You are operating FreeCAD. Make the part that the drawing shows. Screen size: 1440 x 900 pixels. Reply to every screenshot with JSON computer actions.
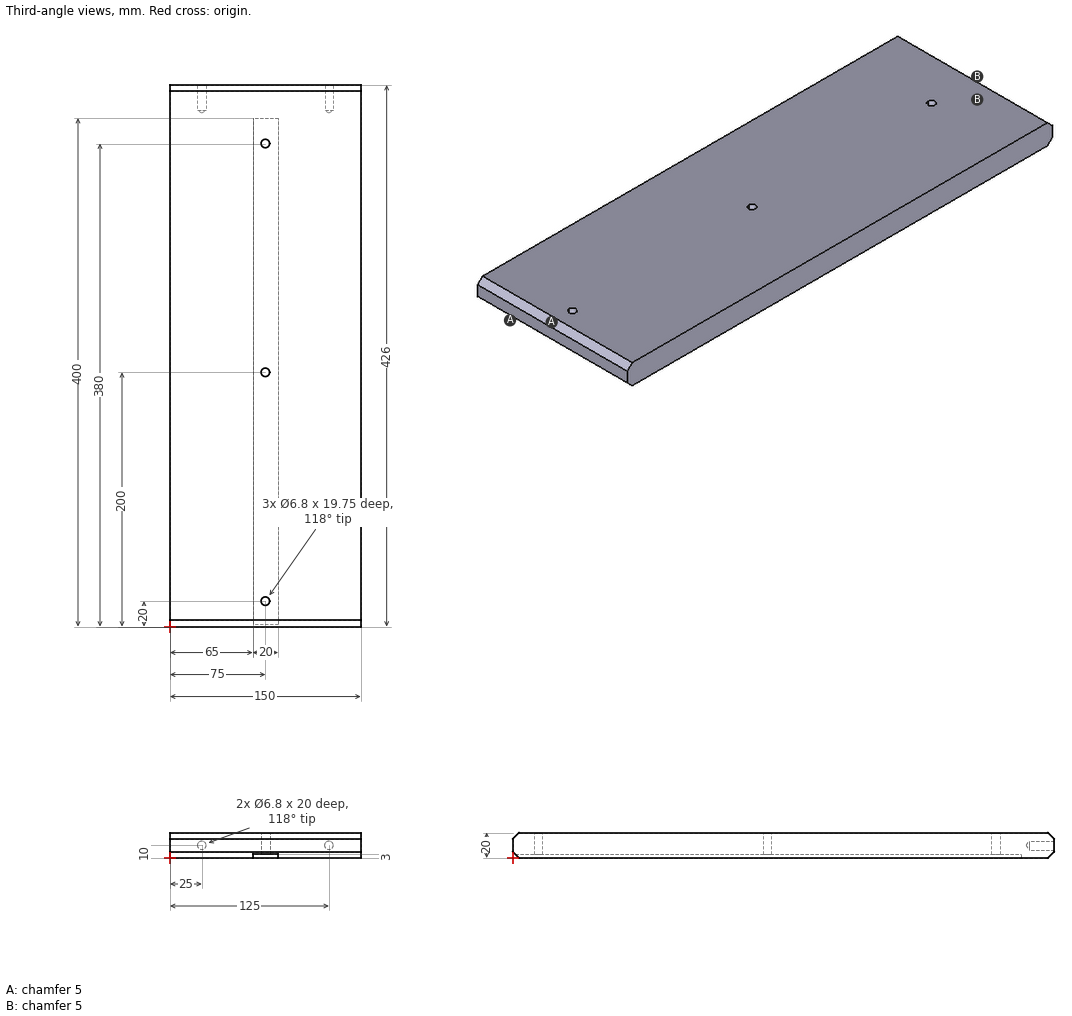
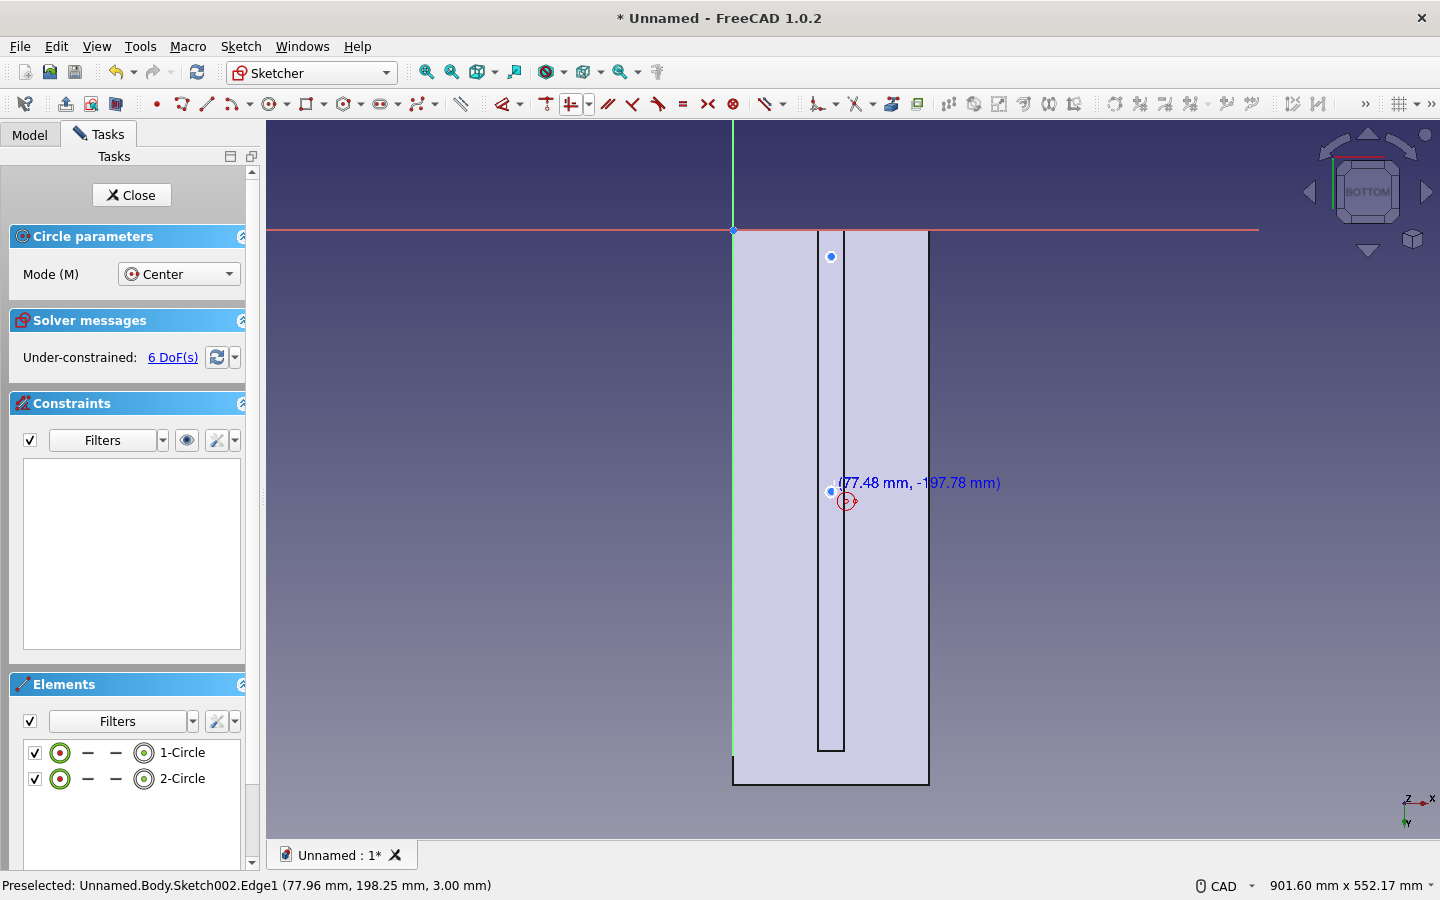
{"action": "scroll", "coordinate": [831, 725], "scroll_direction": "up", "scroll_amount": 9}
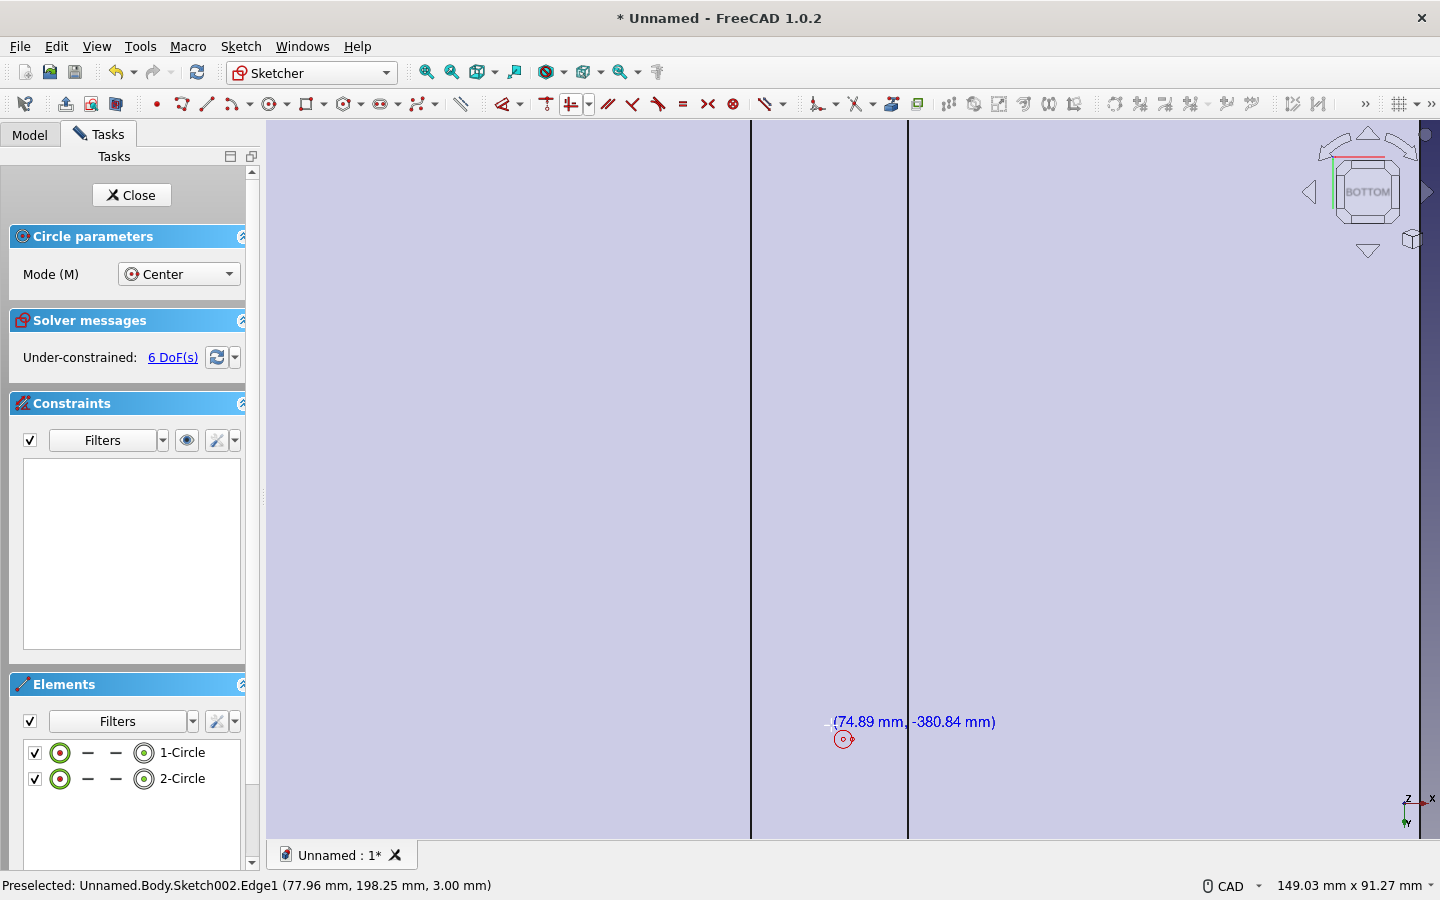
{"action": "scroll", "coordinate": [831, 726], "scroll_direction": "down", "scroll_amount": 9}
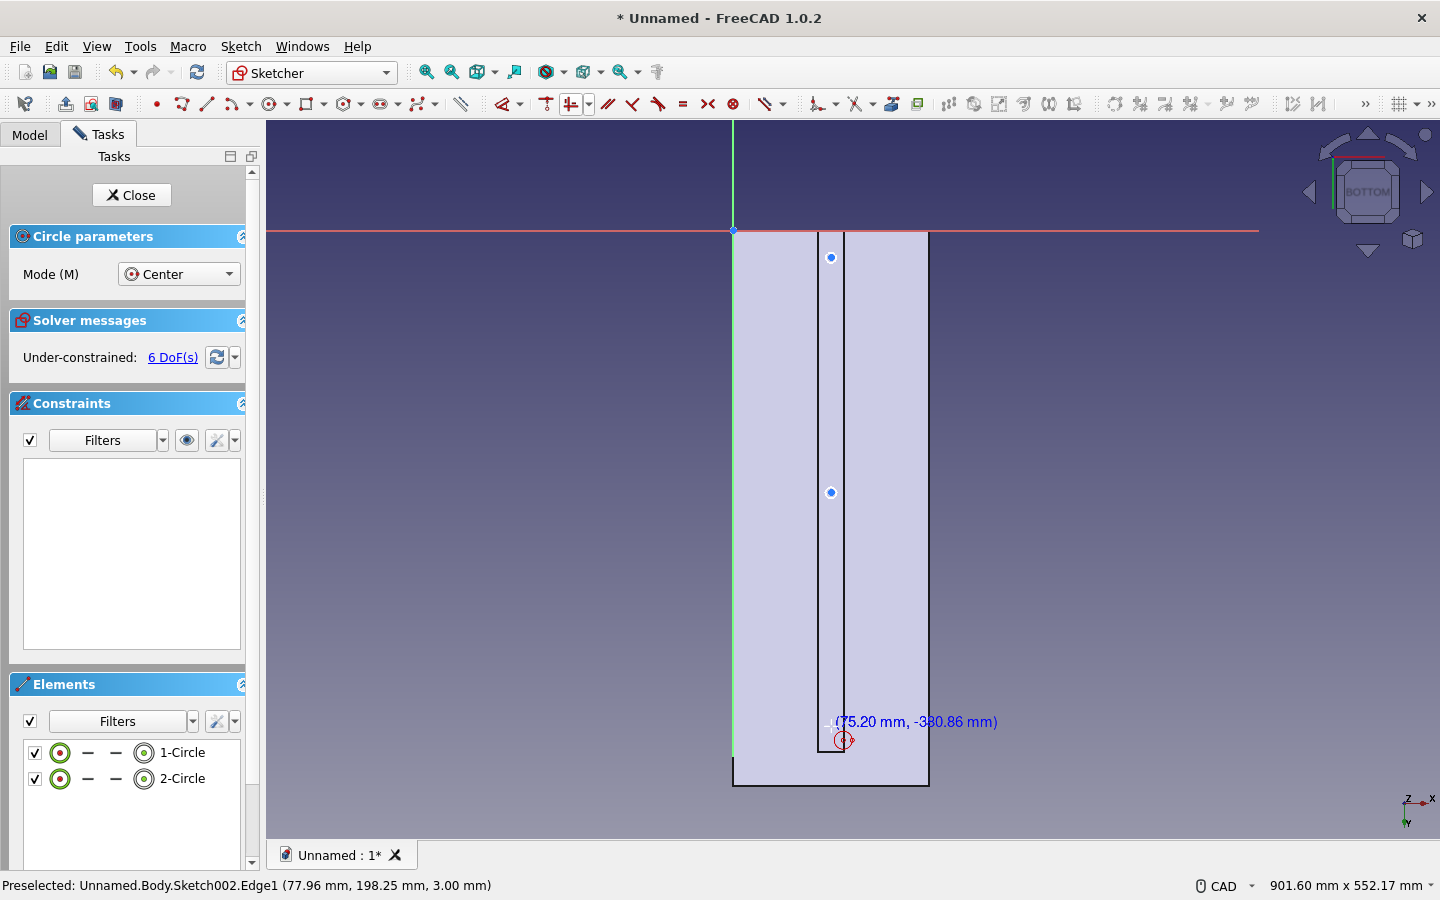
{"action": "left_click", "coordinate": [831, 726]}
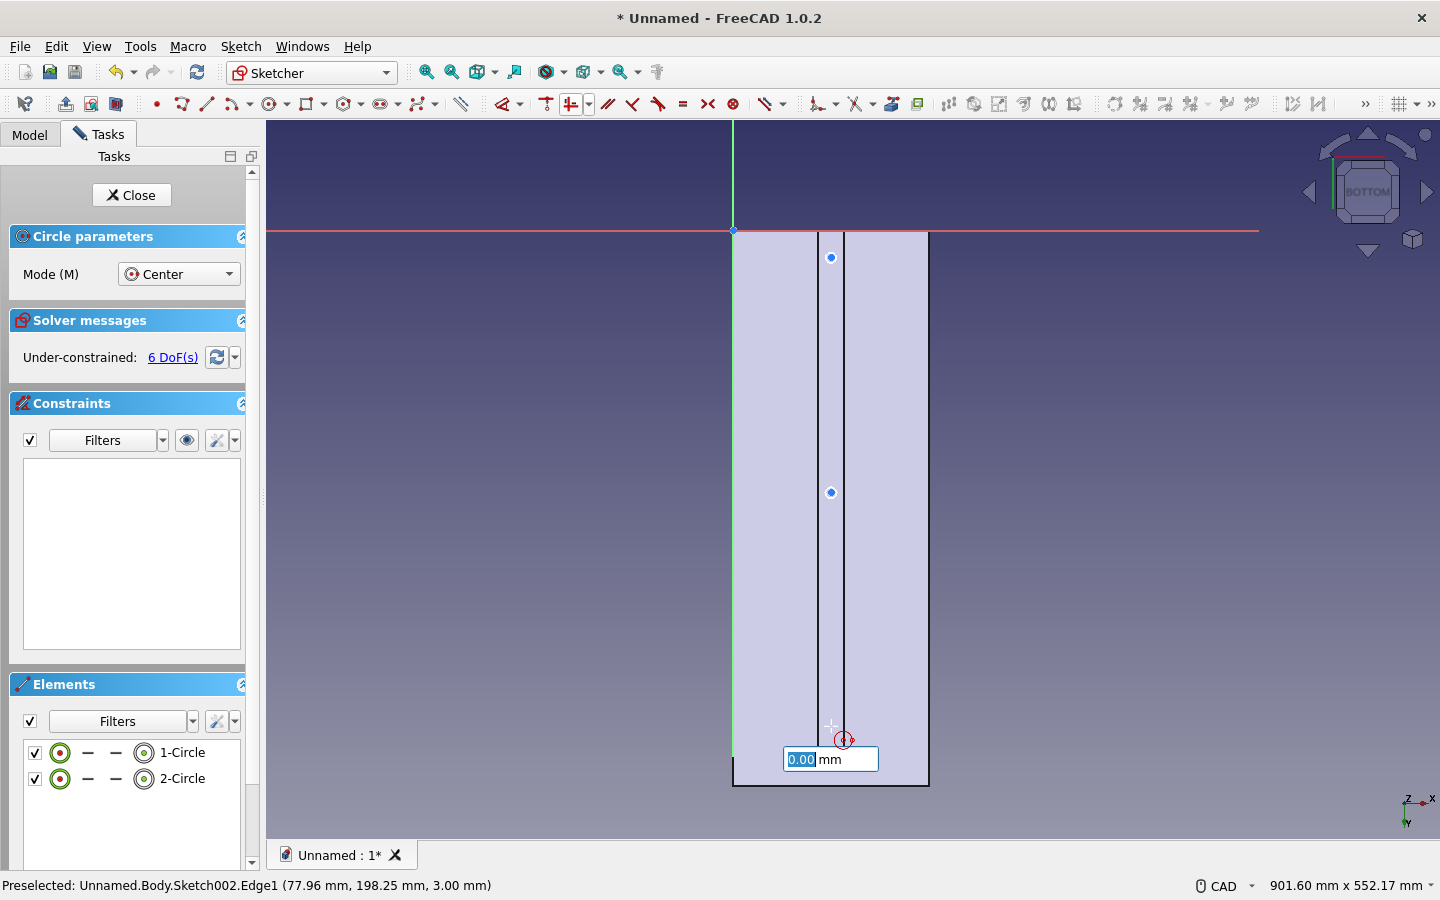
{"action": "scroll", "coordinate": [834, 723], "scroll_direction": "up", "scroll_amount": 7}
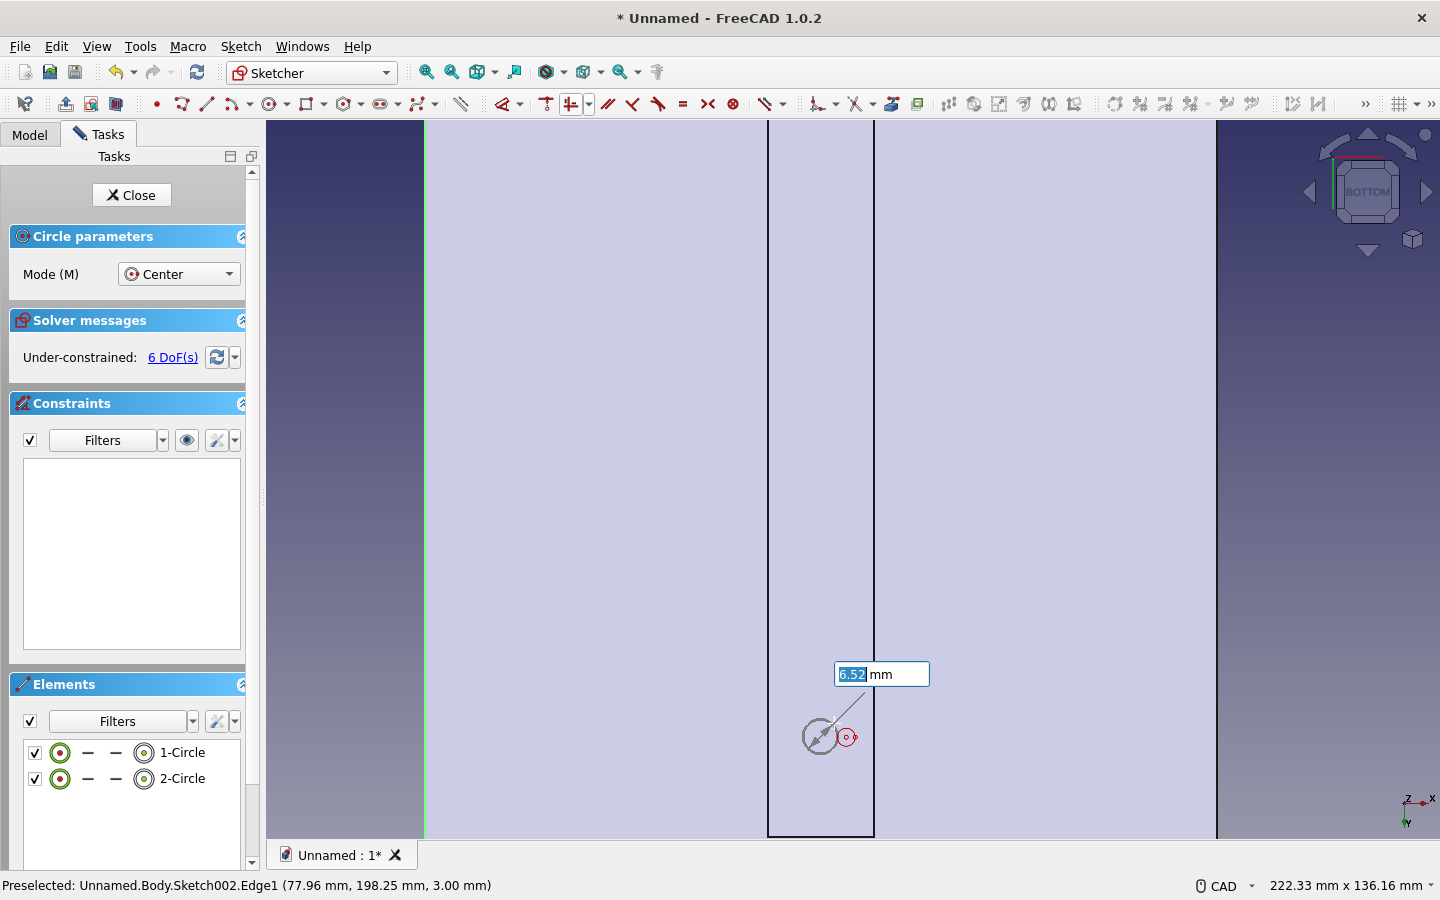
{"action": "left_click", "coordinate": [834, 719]}
{"action": "key", "text": "Escape"}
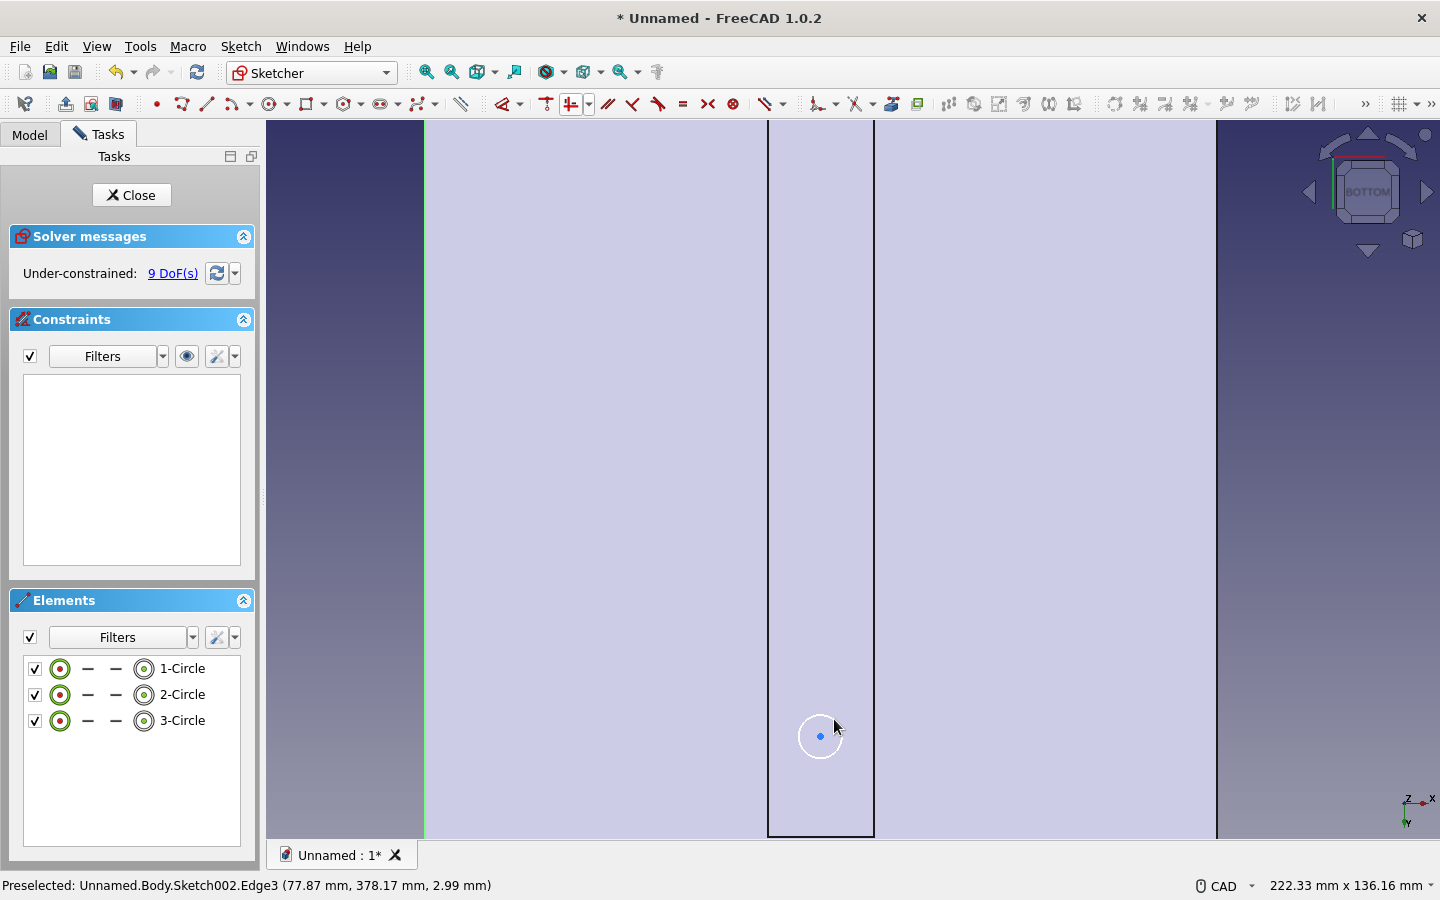
{"action": "scroll", "coordinate": [834, 722], "scroll_direction": "down", "scroll_amount": 7}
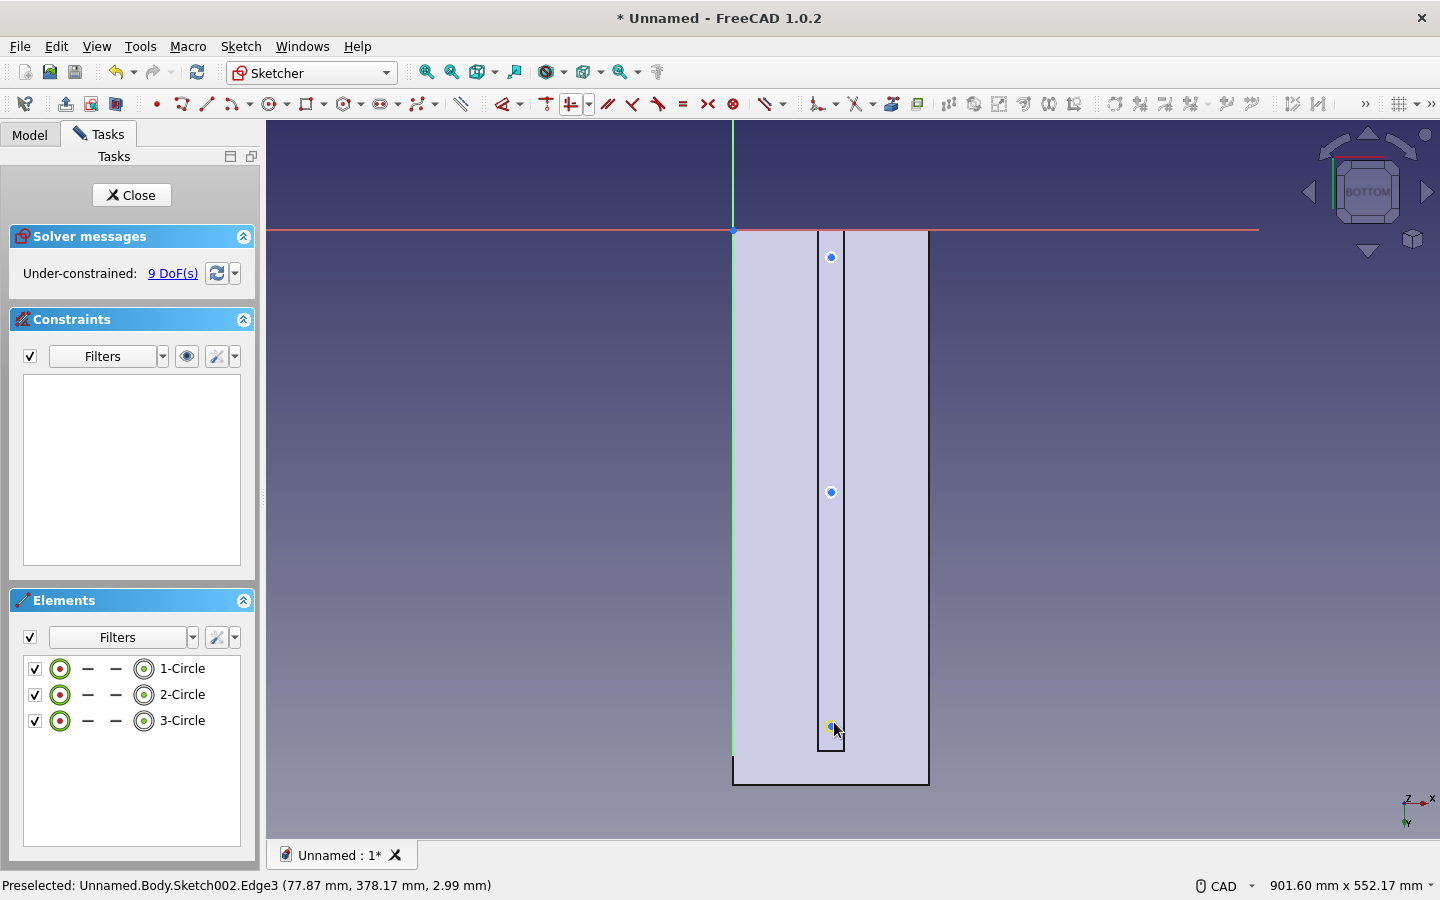
{"action": "scroll", "coordinate": [835, 253], "scroll_direction": "up", "scroll_amount": 5}